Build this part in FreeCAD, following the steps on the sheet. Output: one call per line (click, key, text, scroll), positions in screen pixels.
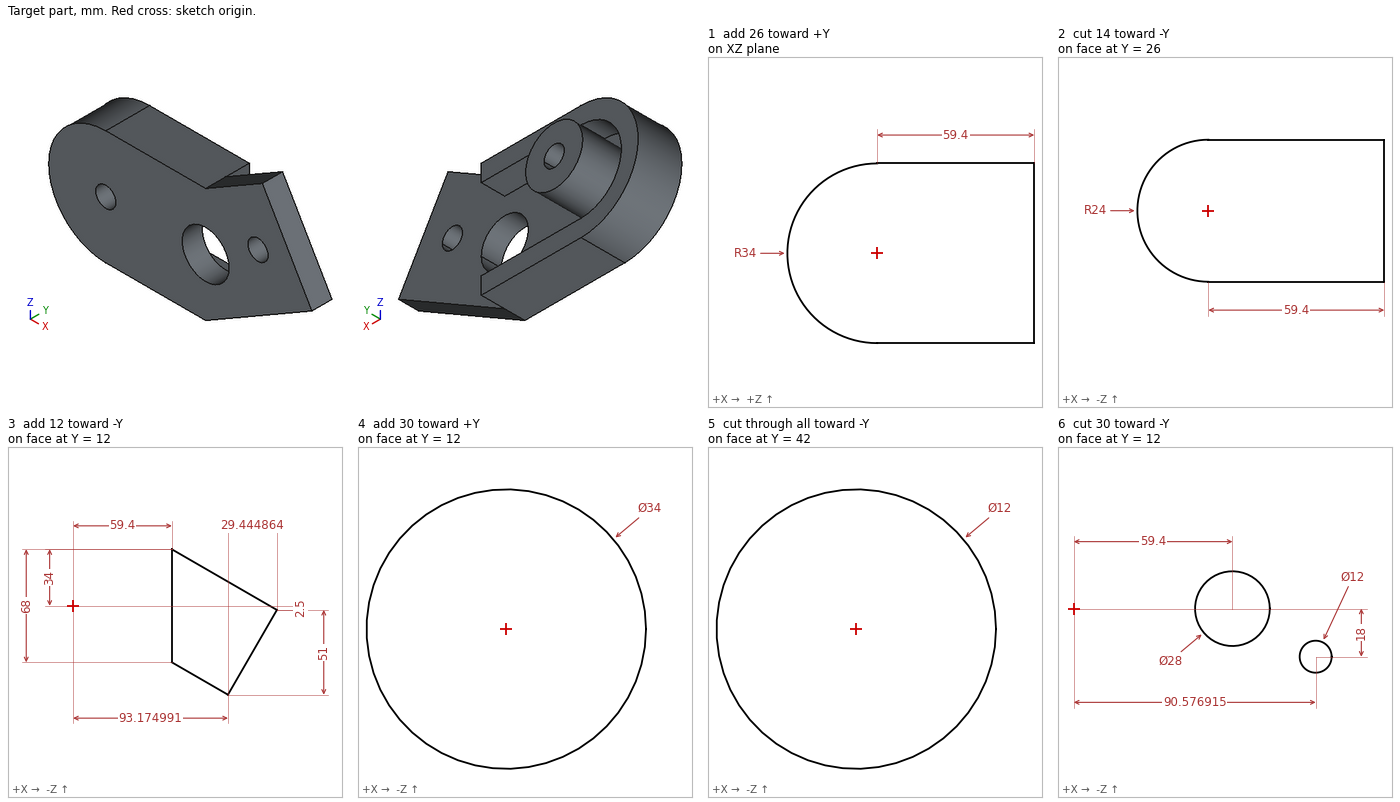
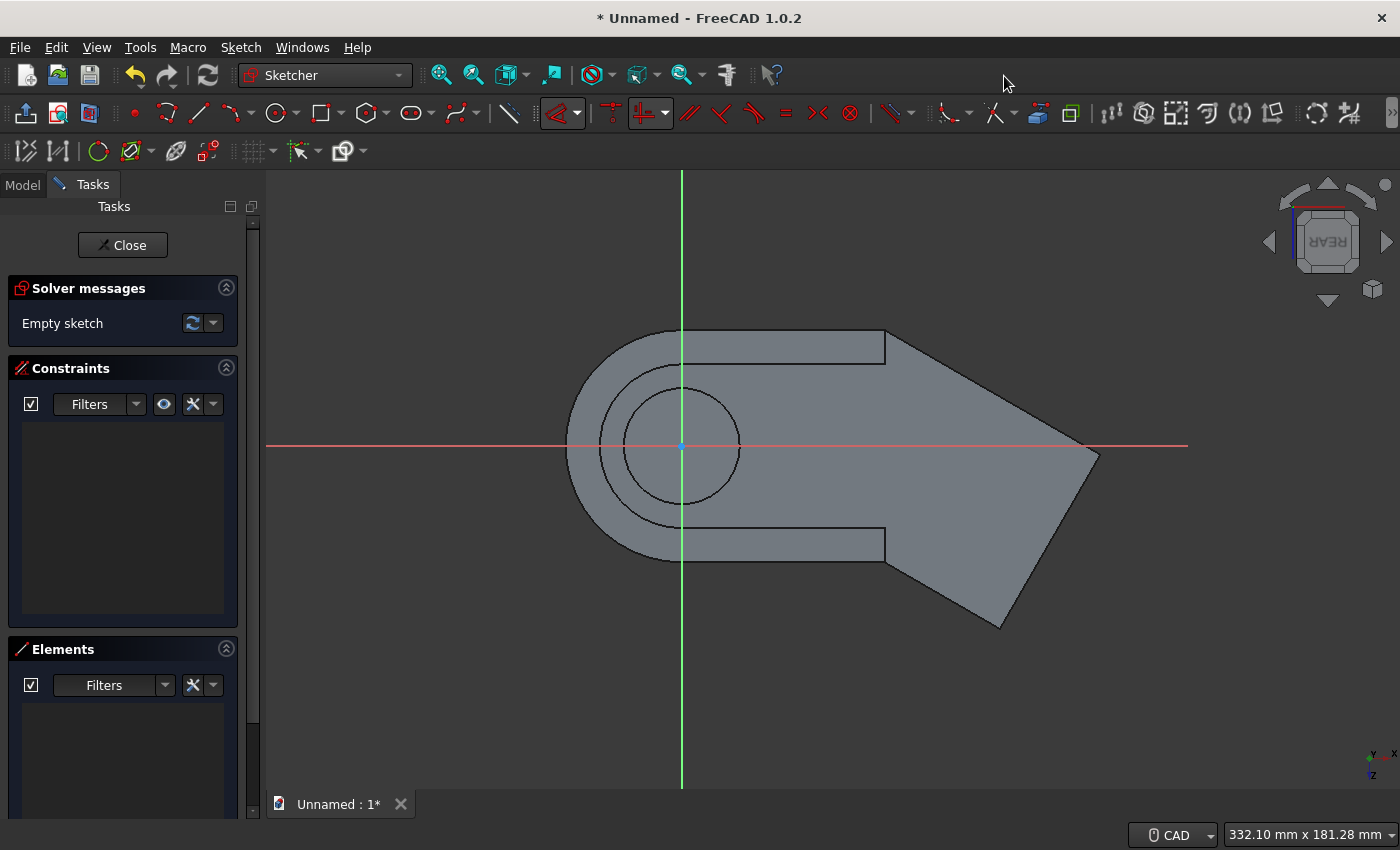
scroll(671, 442, up, 11)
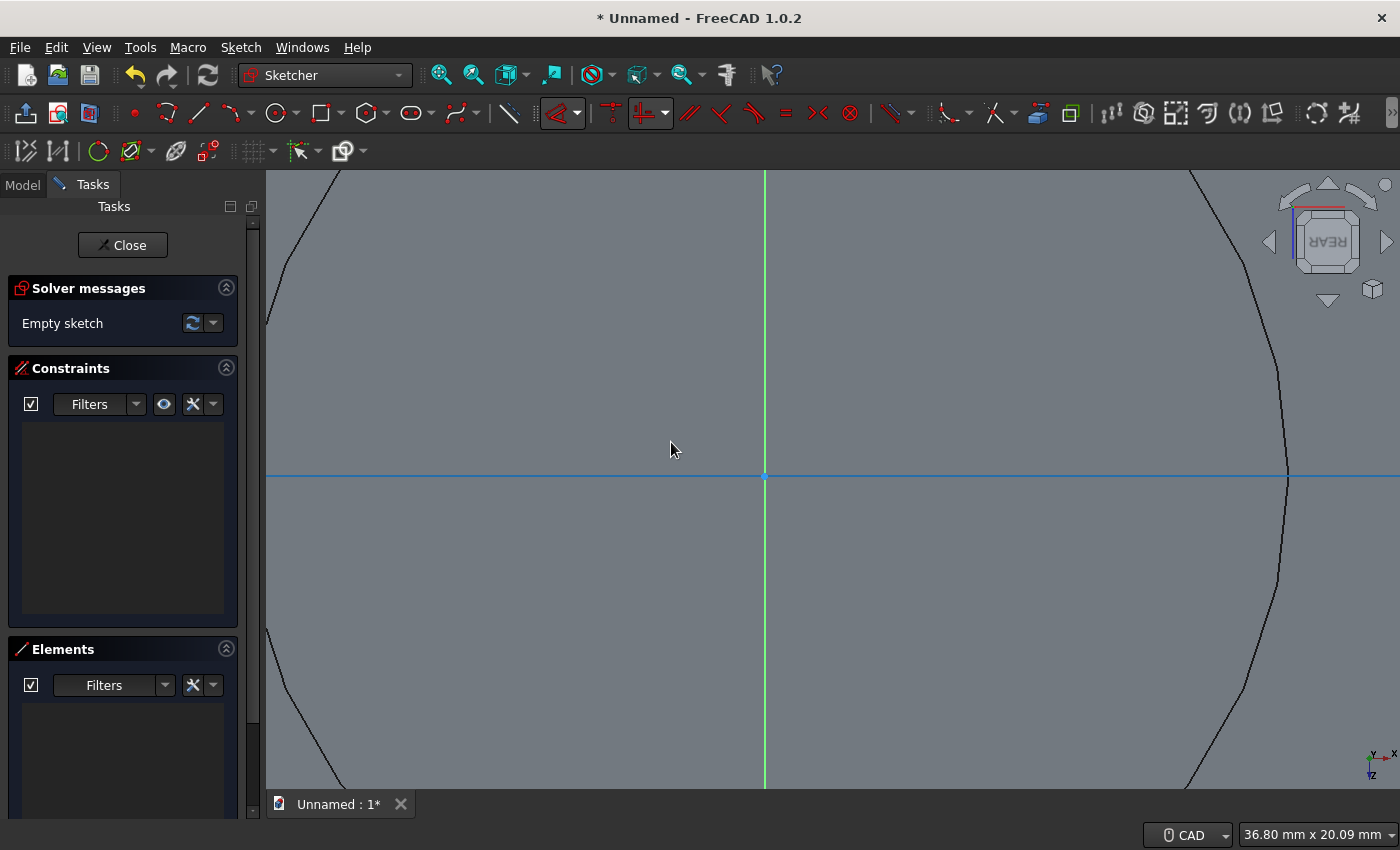
click(276, 114)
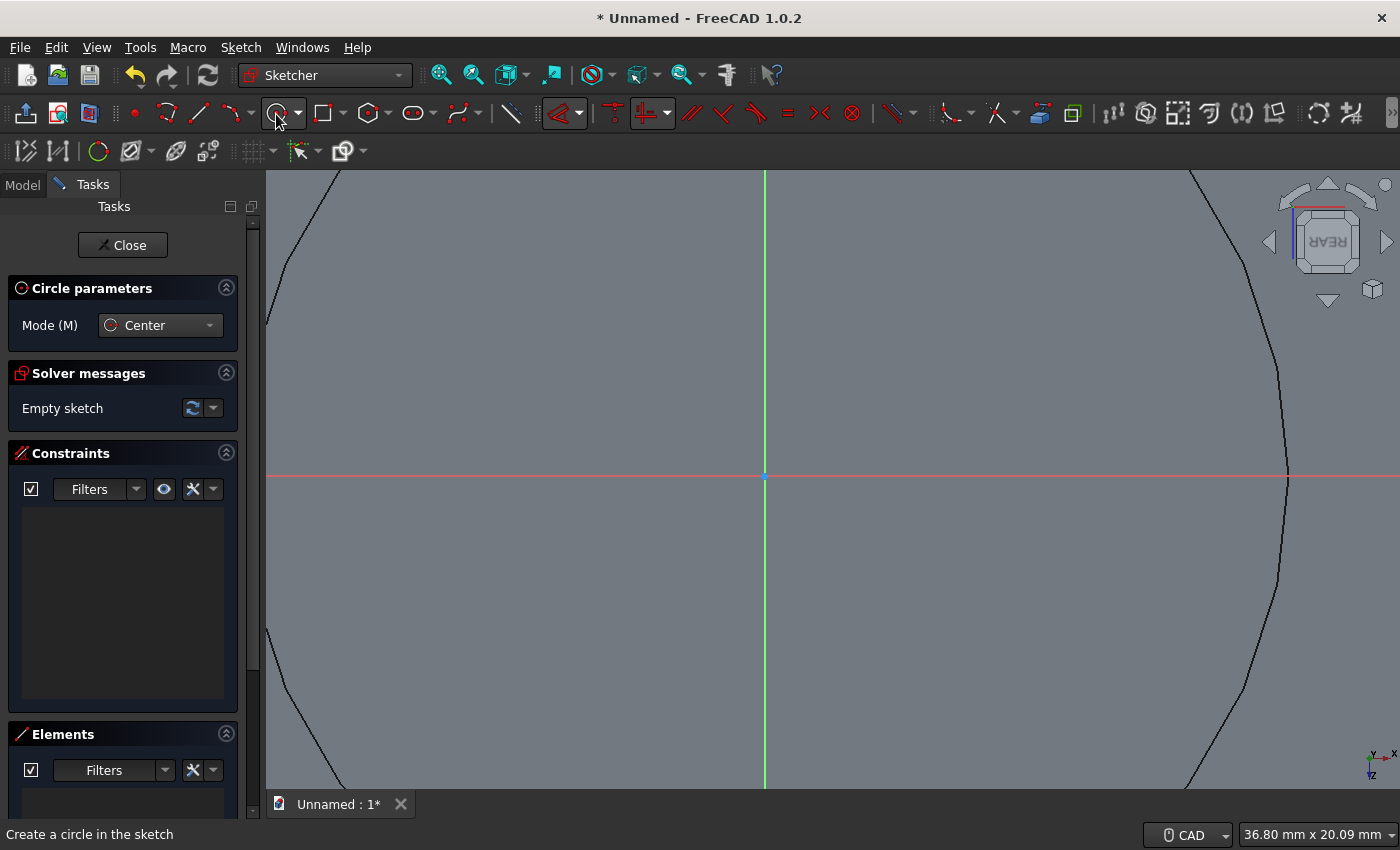
click(765, 476)
move(895, 346)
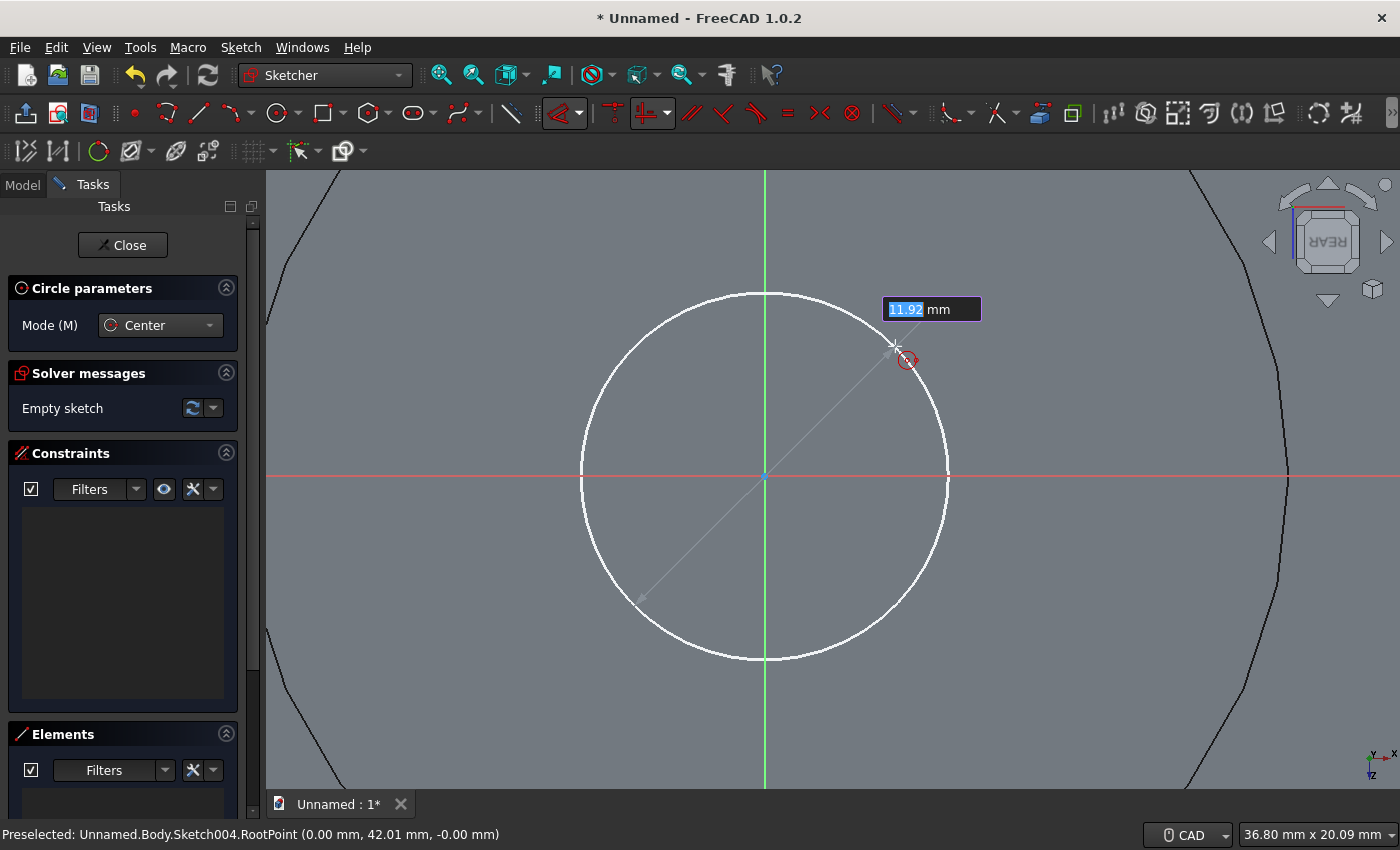
text(12)
key(Return)
key(Escape)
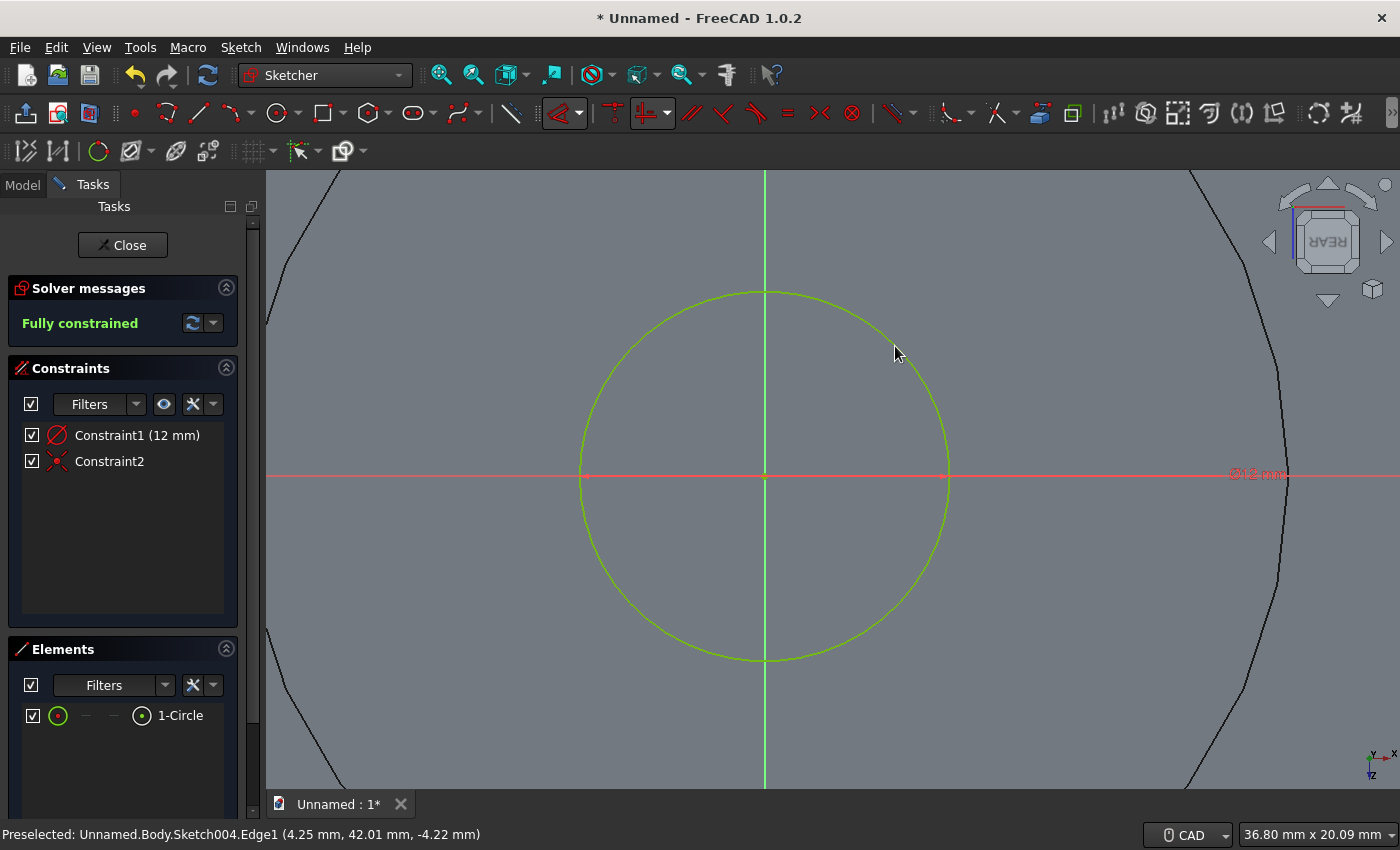
click(123, 245)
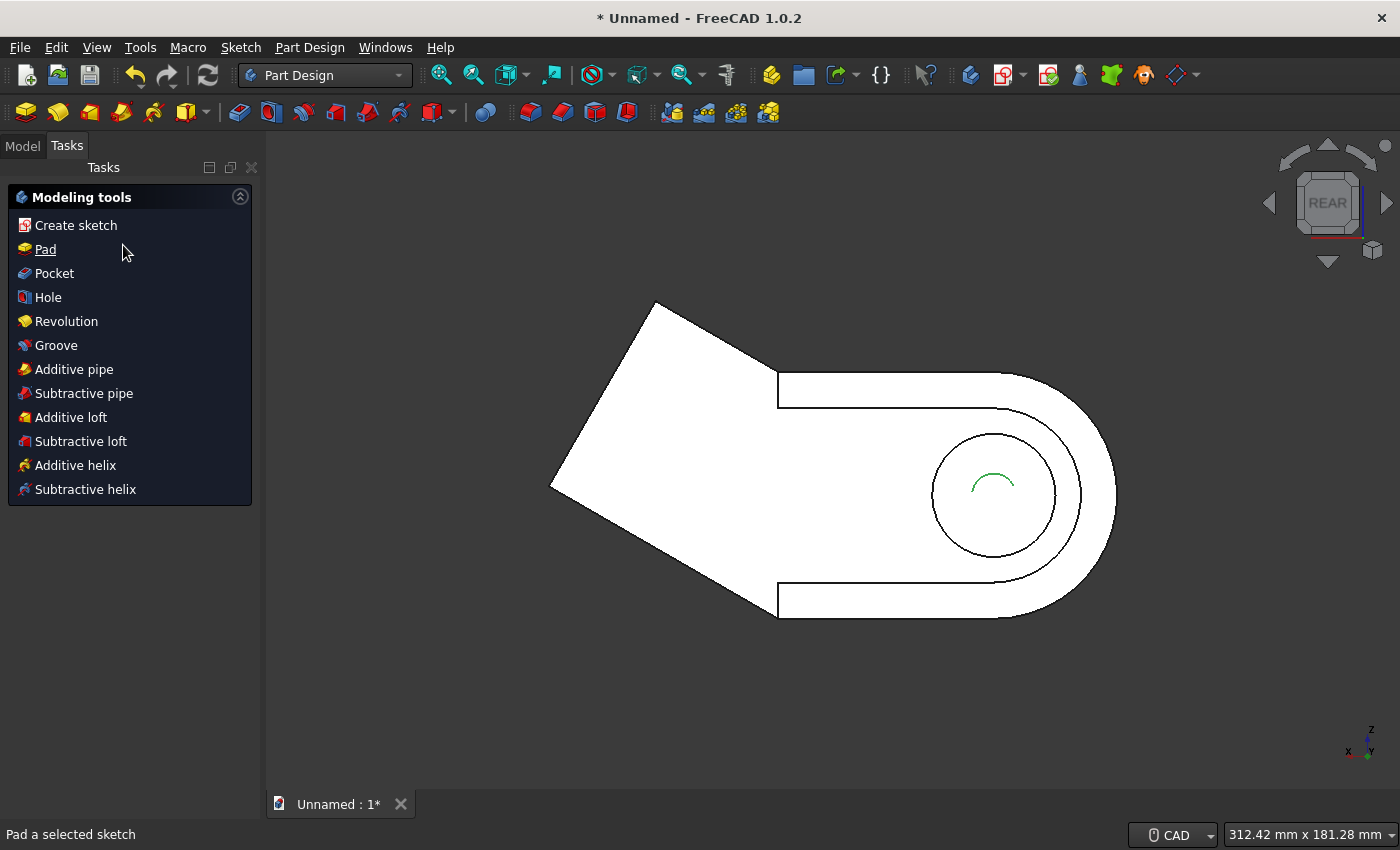
click(240, 112)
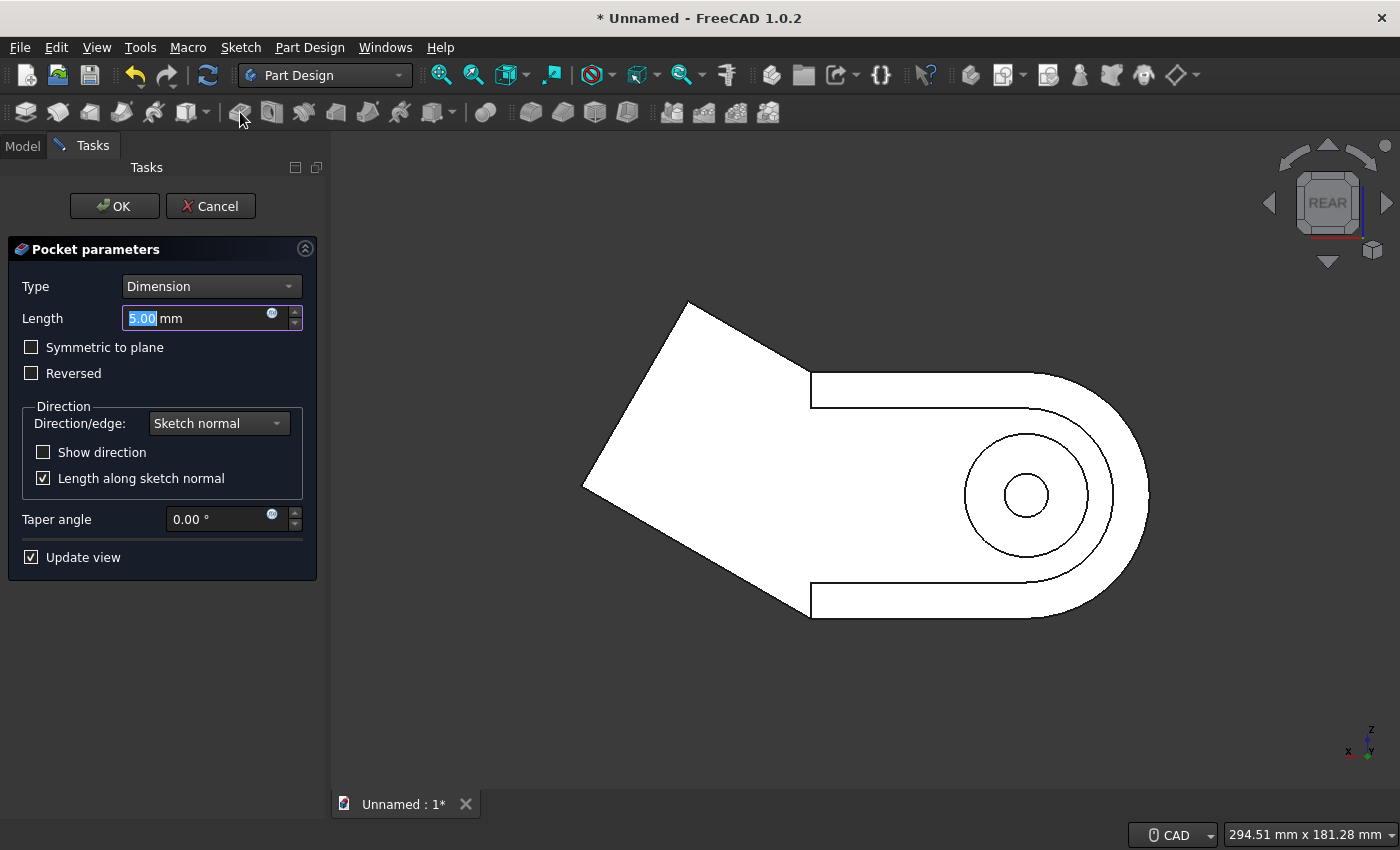
click(212, 286)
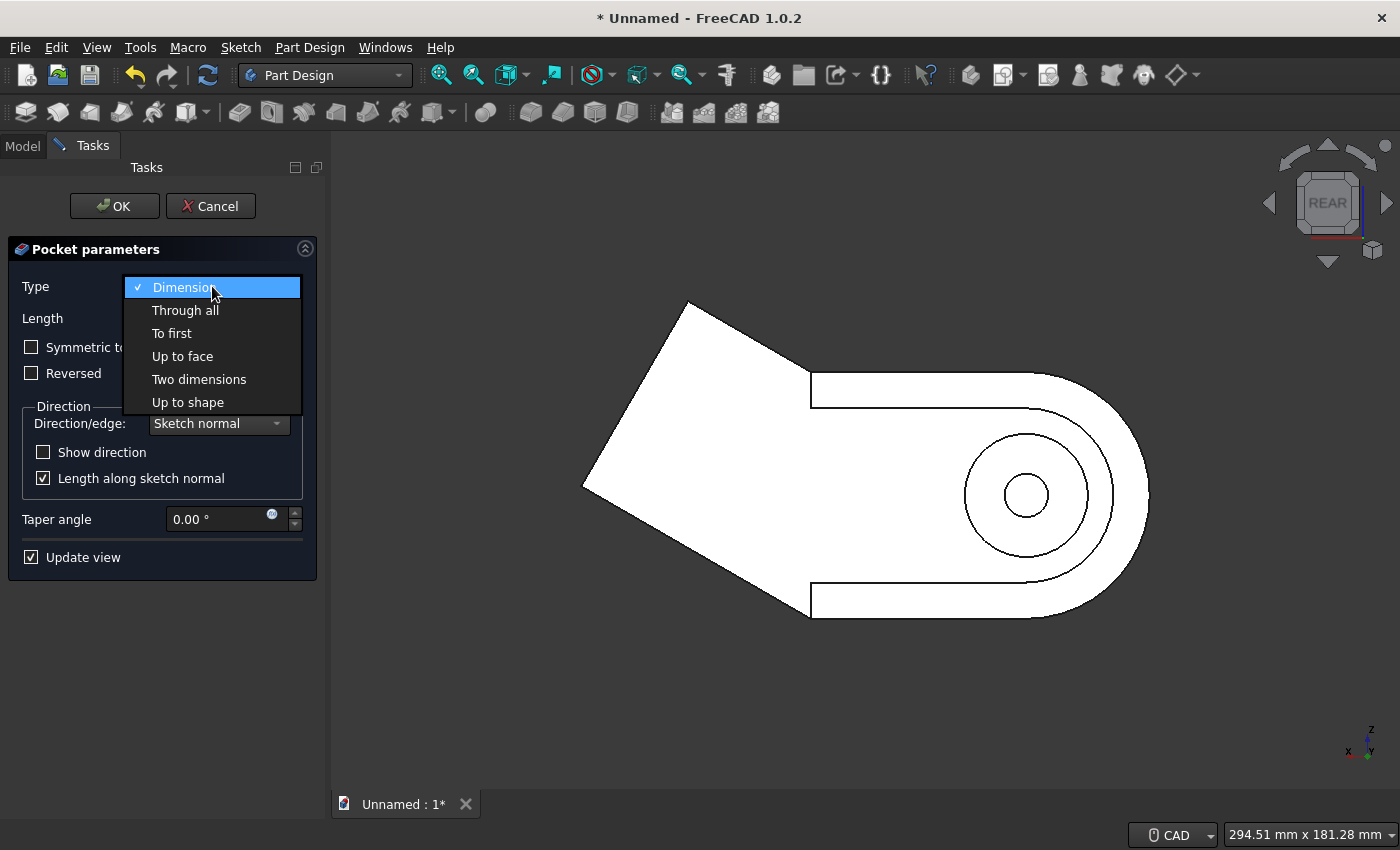
click(212, 310)